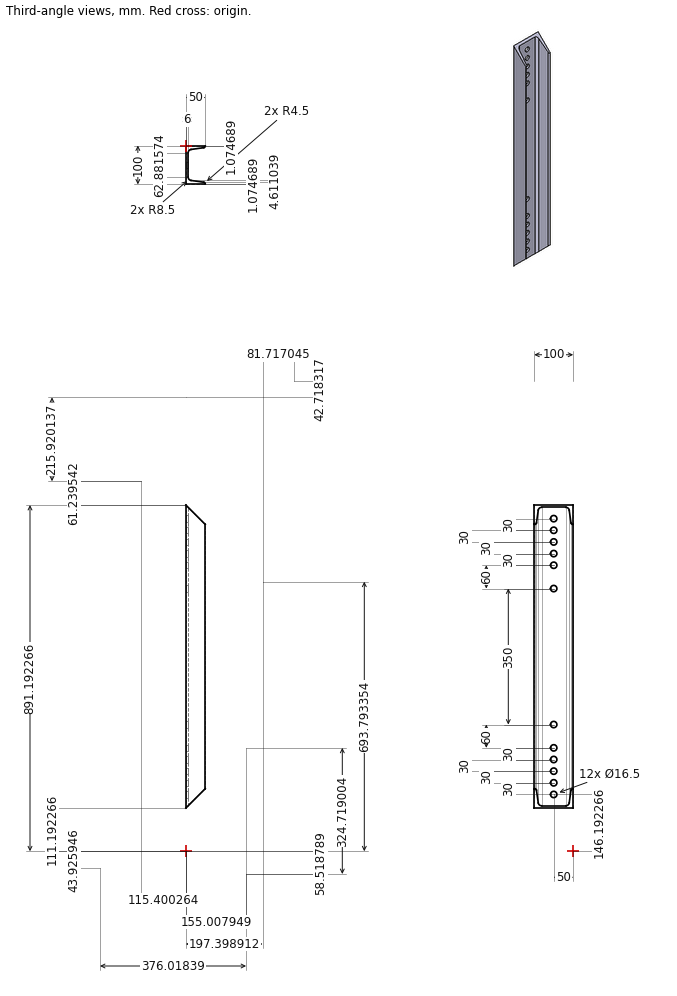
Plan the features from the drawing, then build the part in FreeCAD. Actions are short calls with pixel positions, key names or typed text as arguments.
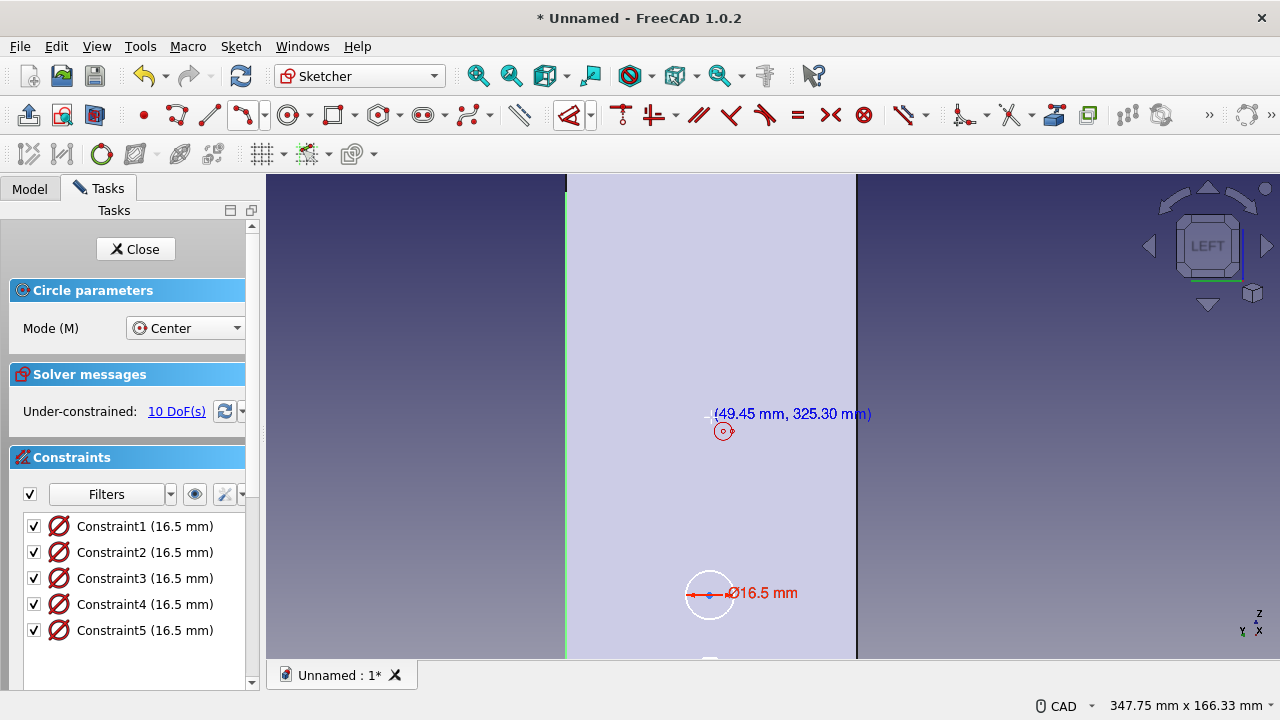
scroll(711, 455, down, 11)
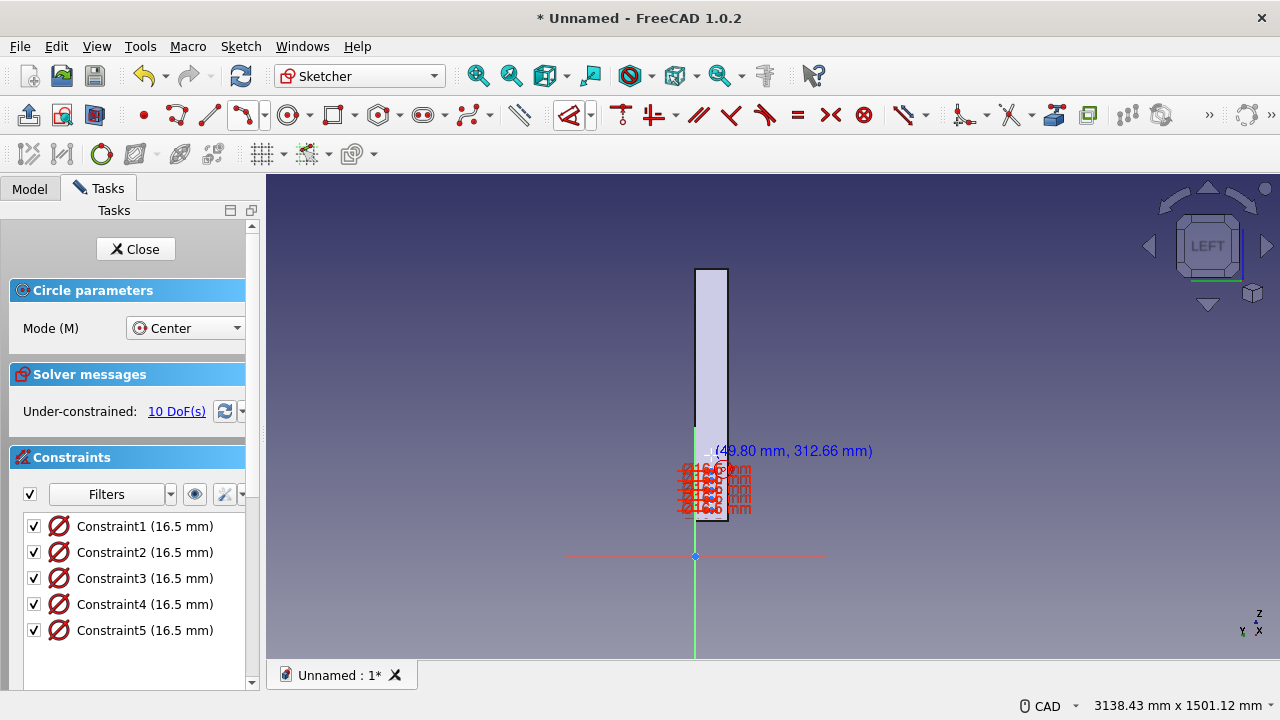
click(711, 451)
move(713, 449)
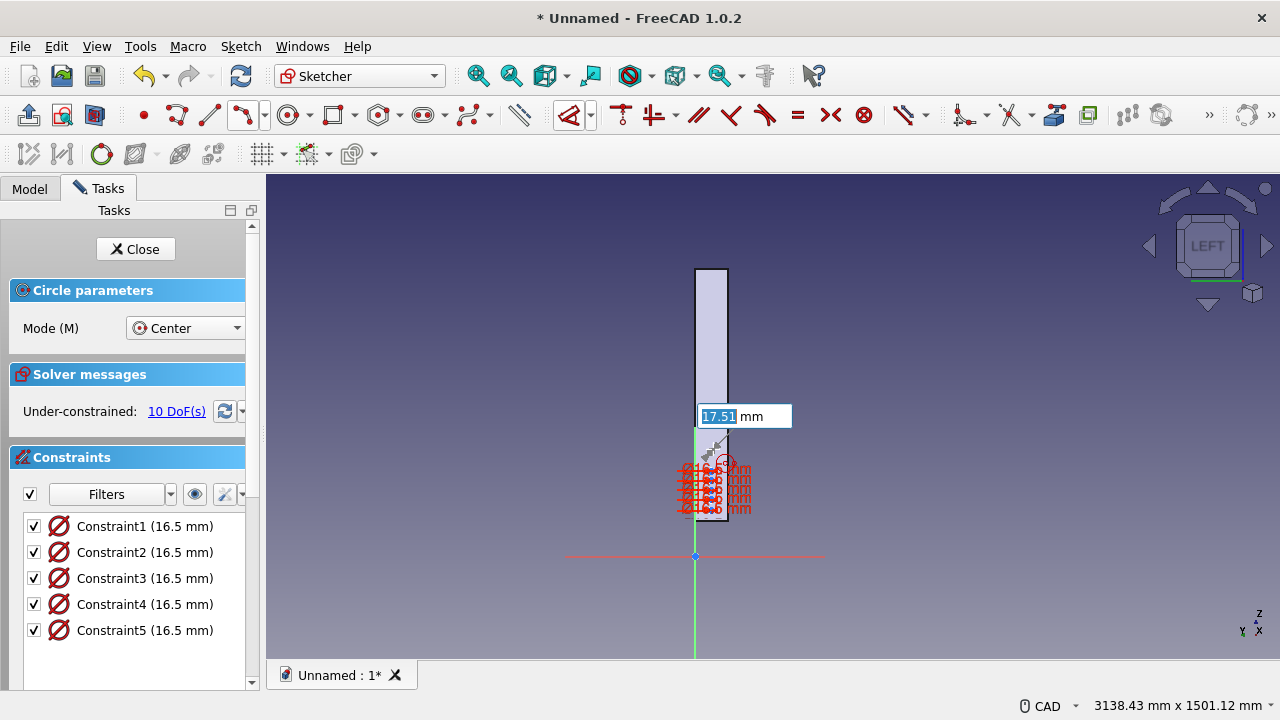
text(16.5)
key(Return)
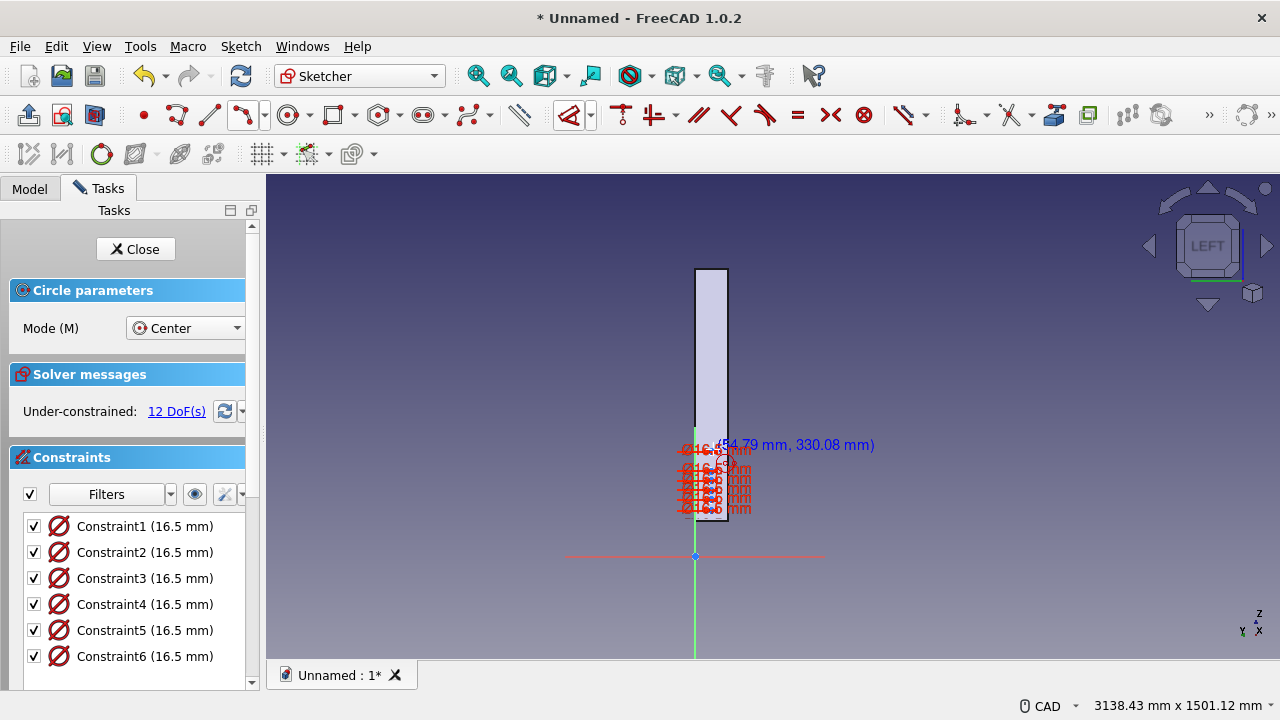
scroll(711, 338, up, 11)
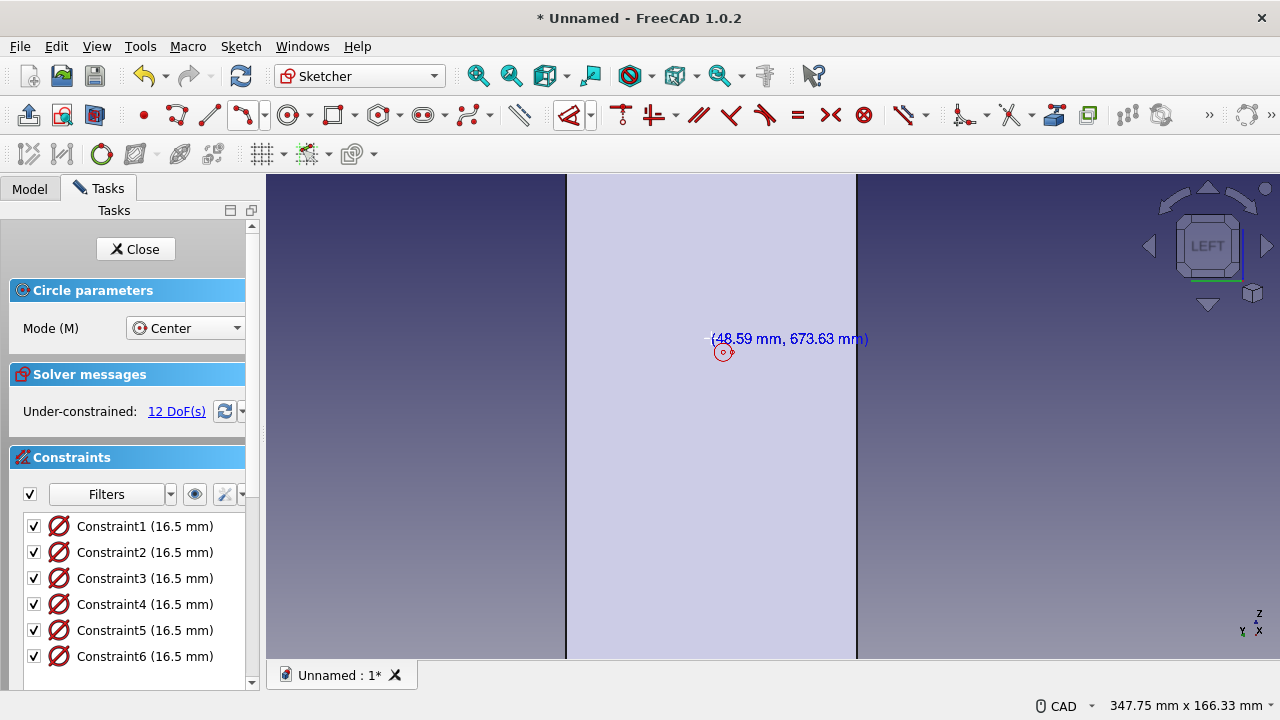
scroll(711, 338, down, 11)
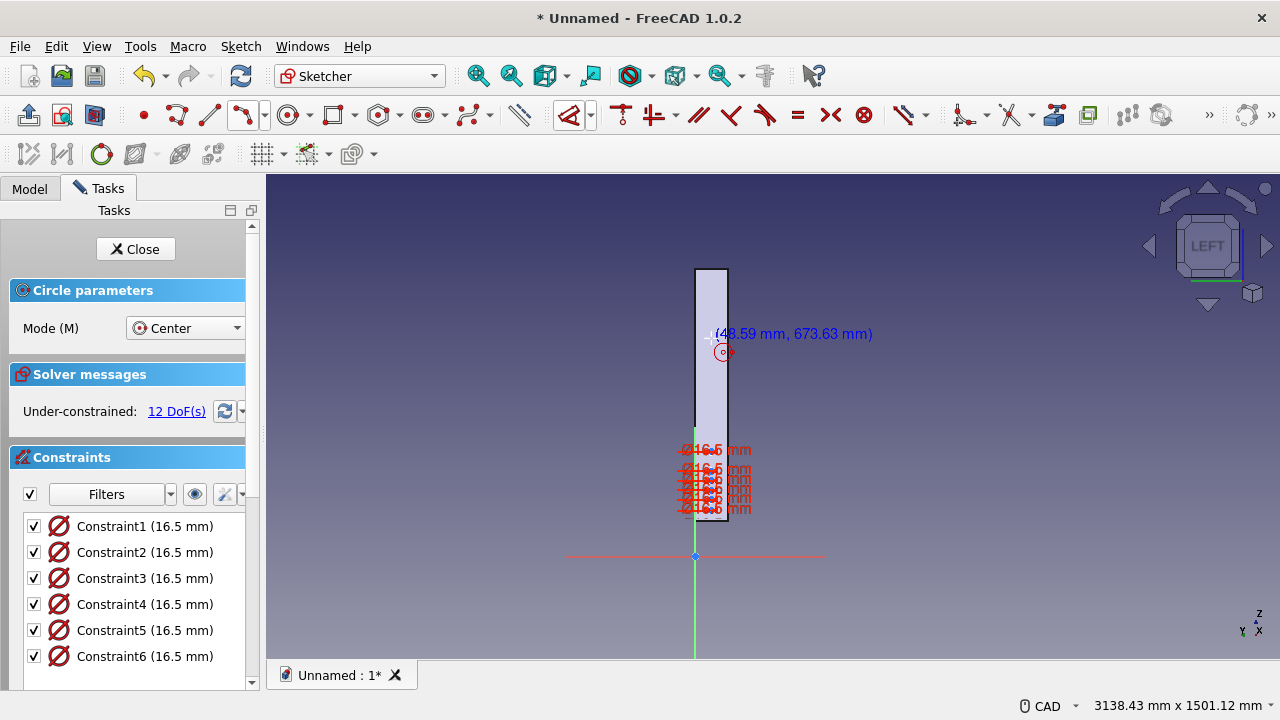
click(711, 338)
move(713, 336)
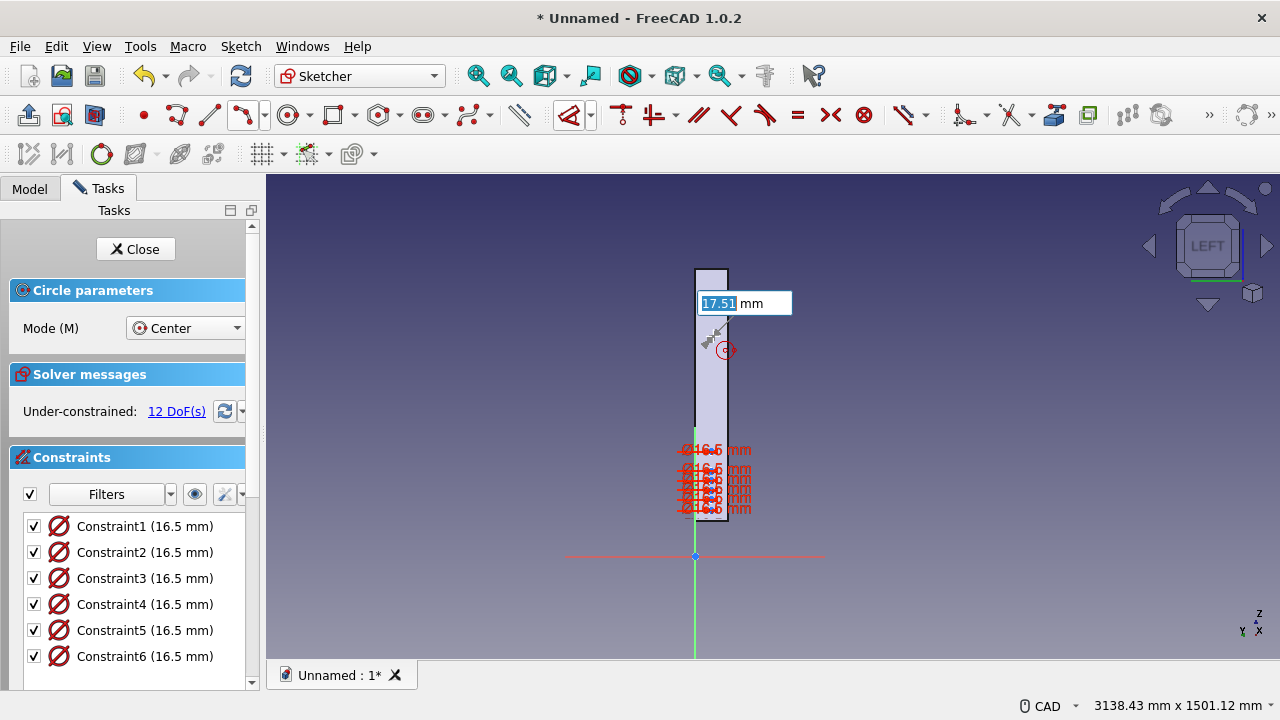
text(16.5)
key(Return)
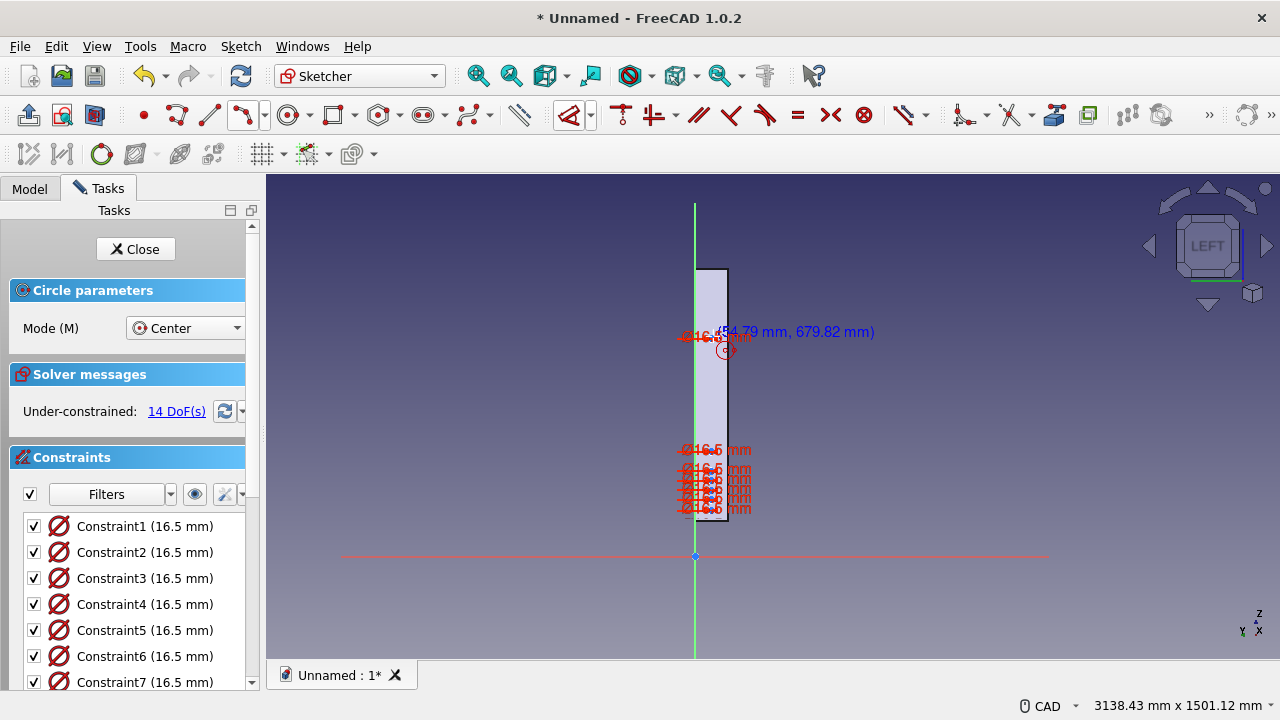
scroll(711, 319, up, 11)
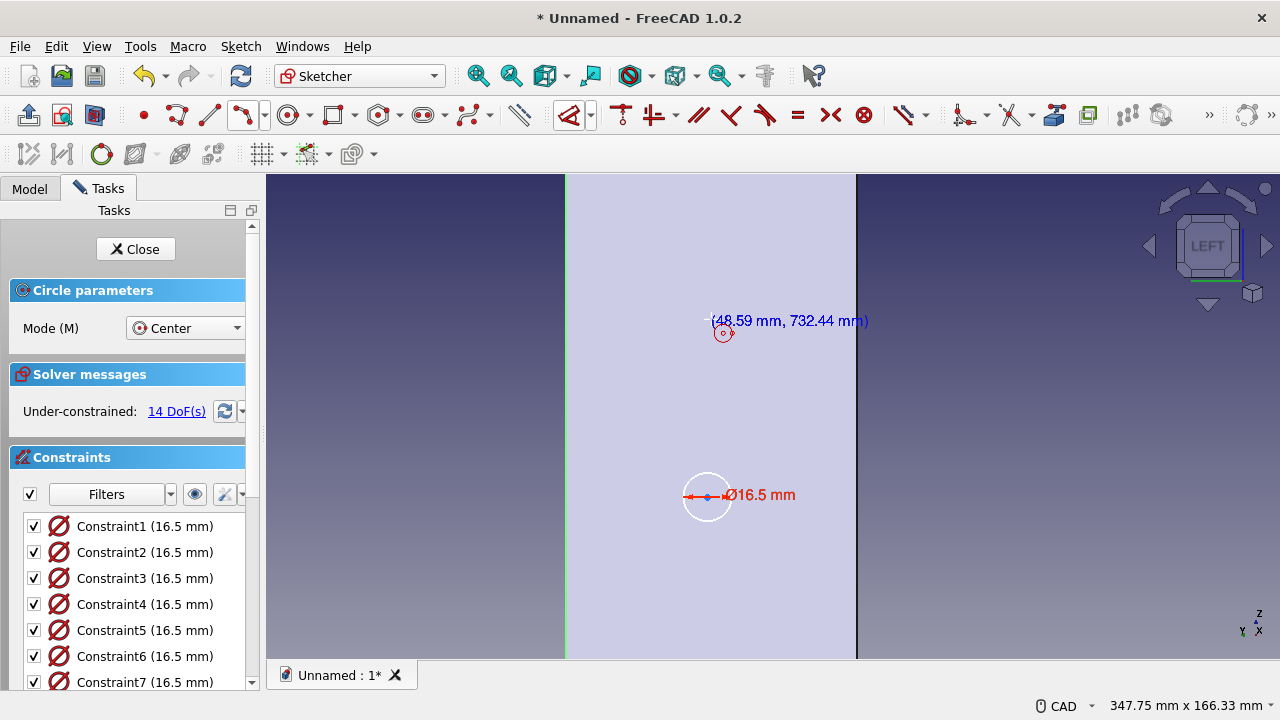
scroll(711, 319, down, 11)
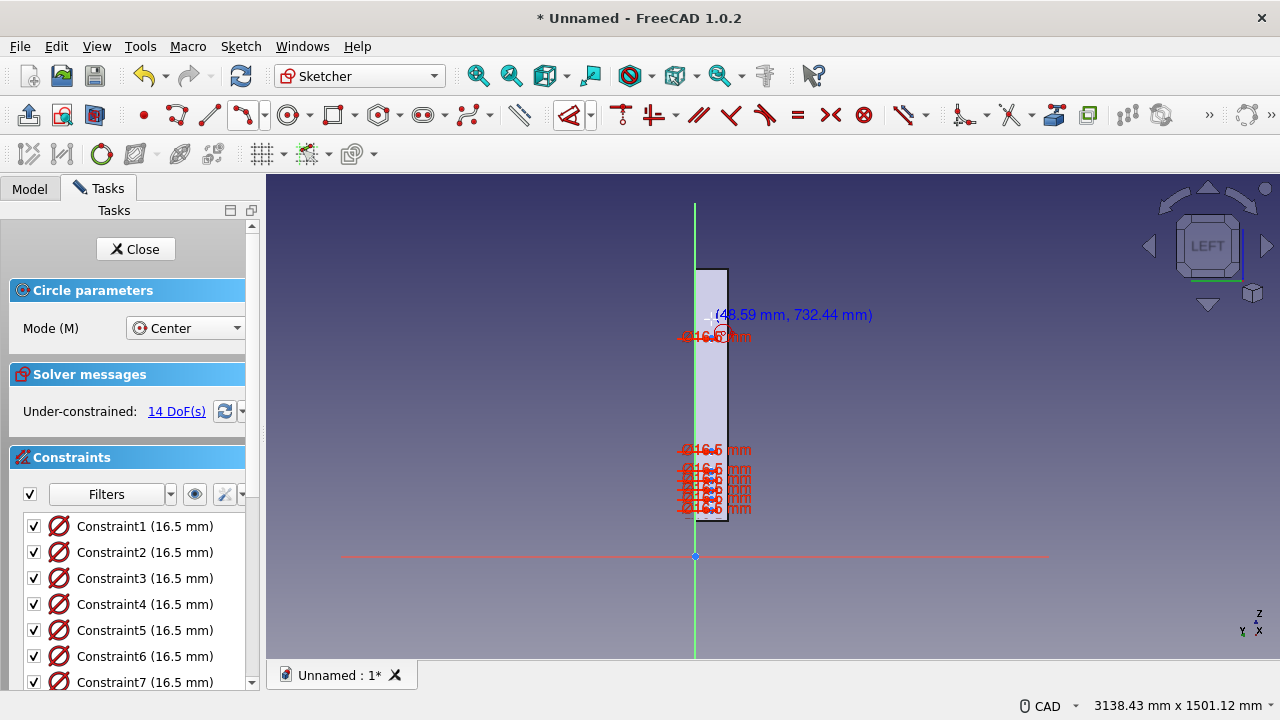
click(711, 319)
move(713, 317)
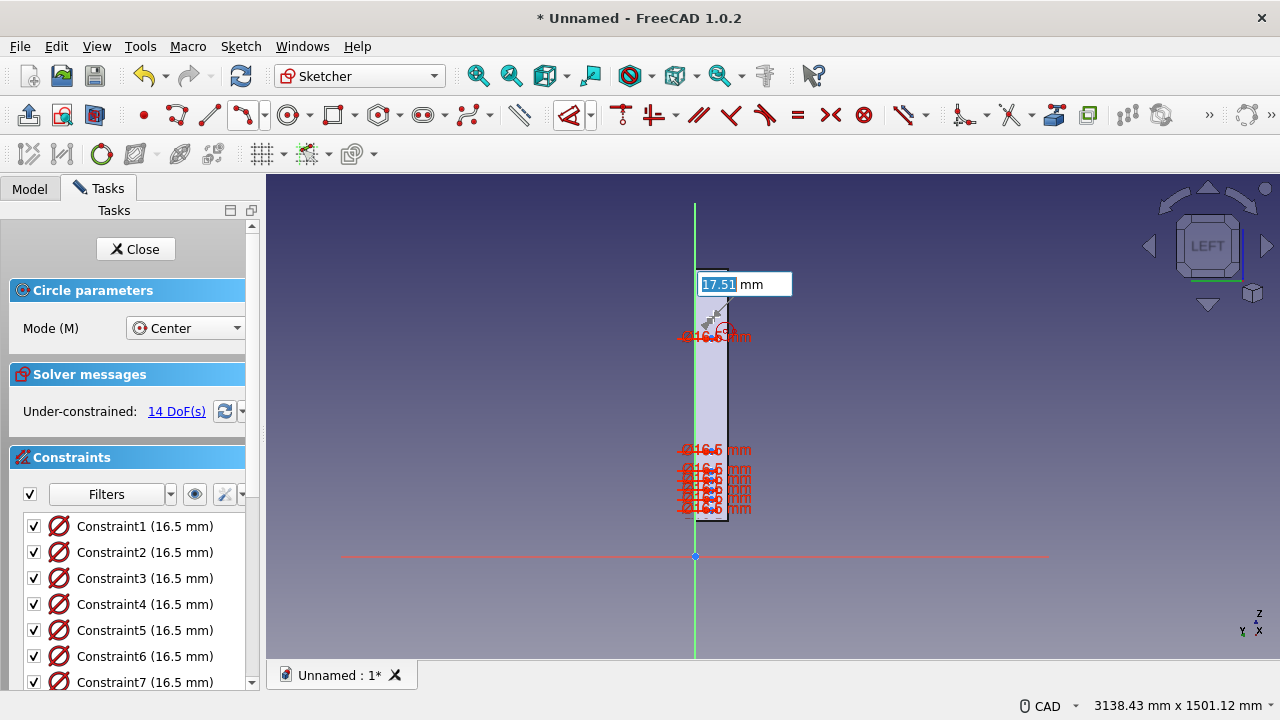
text(16.5)
key(Return)